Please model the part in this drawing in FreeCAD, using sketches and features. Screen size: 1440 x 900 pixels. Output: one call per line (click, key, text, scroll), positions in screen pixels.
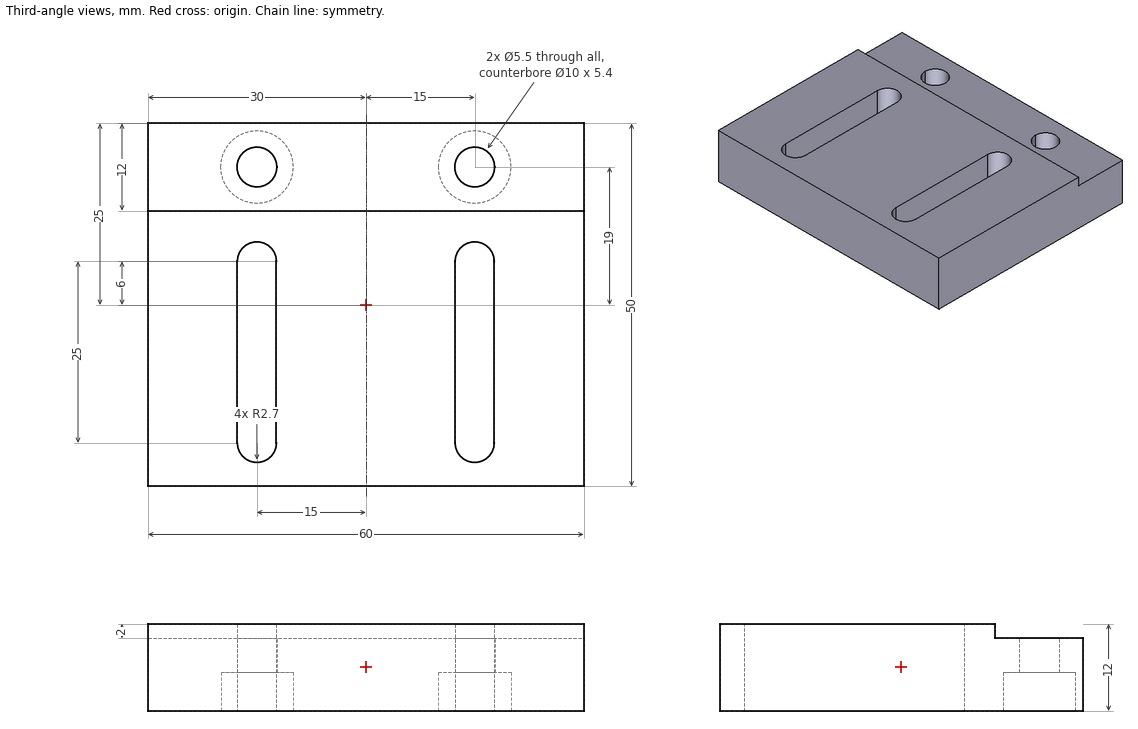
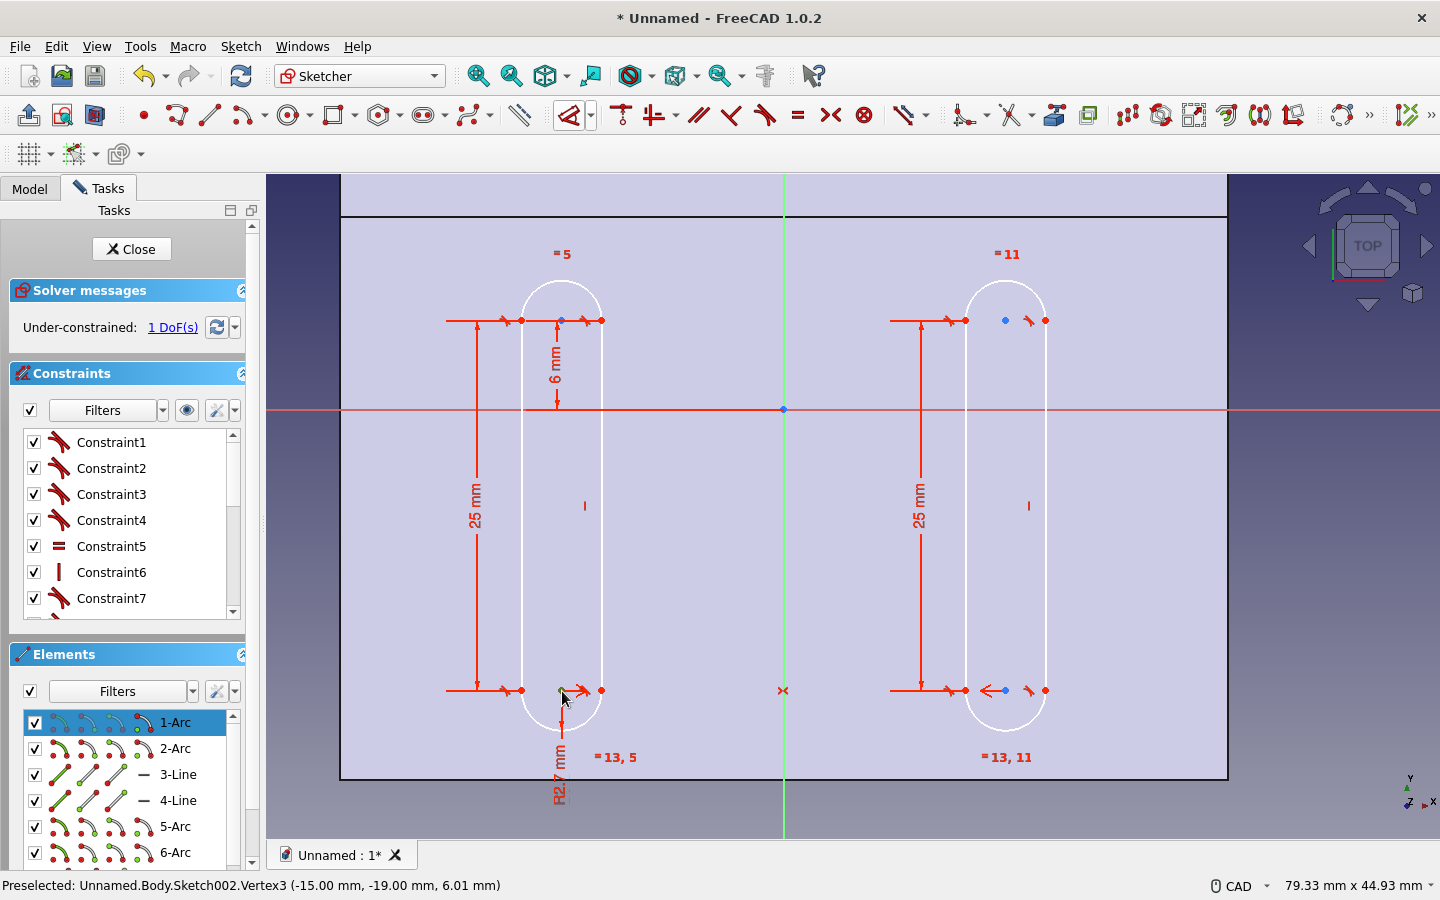
key(l)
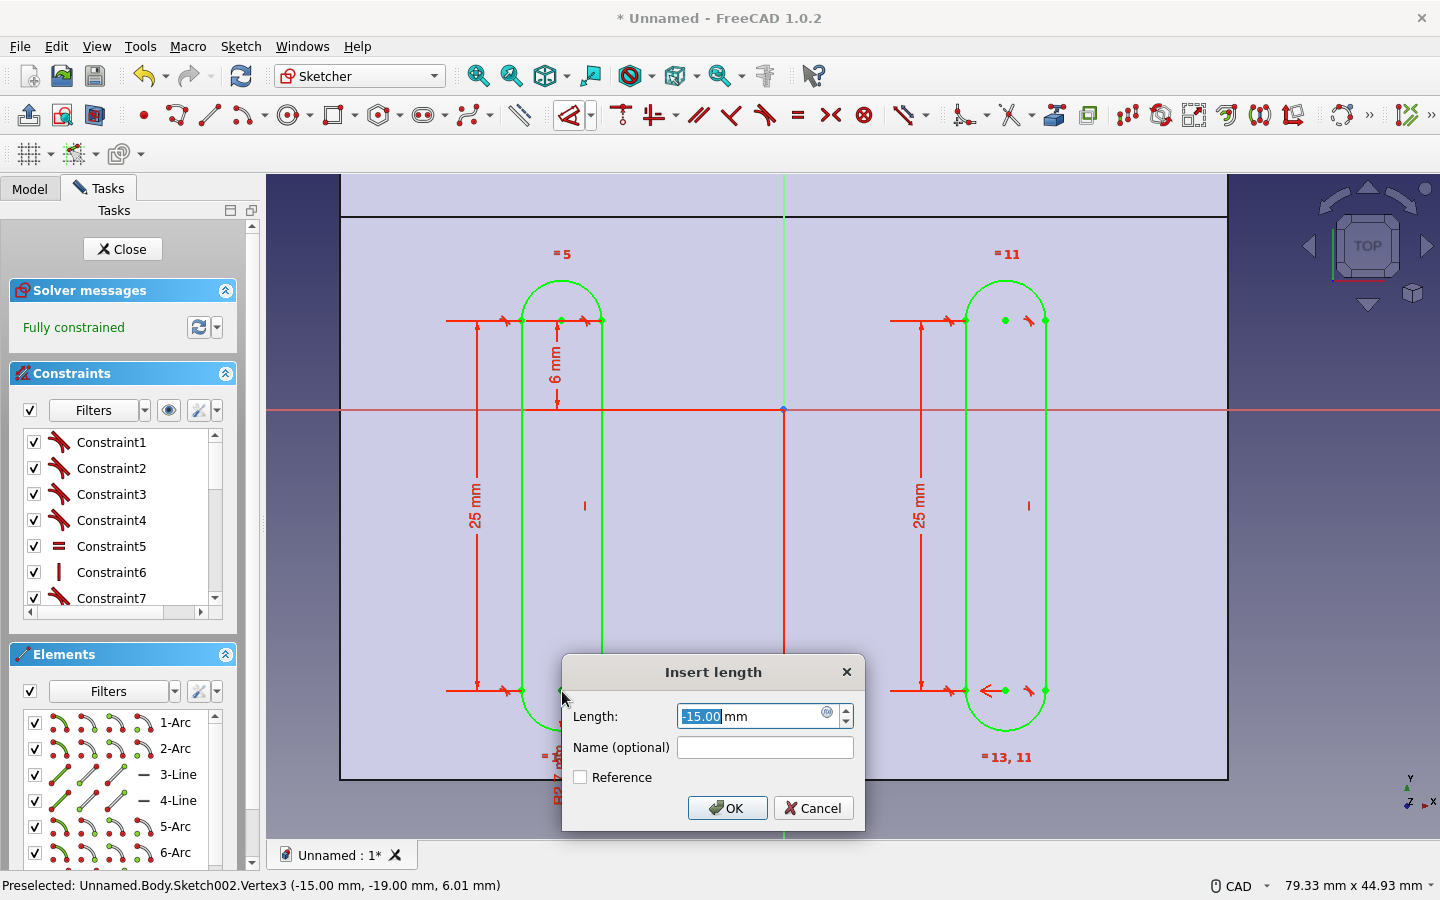
text(-15)
key(Return)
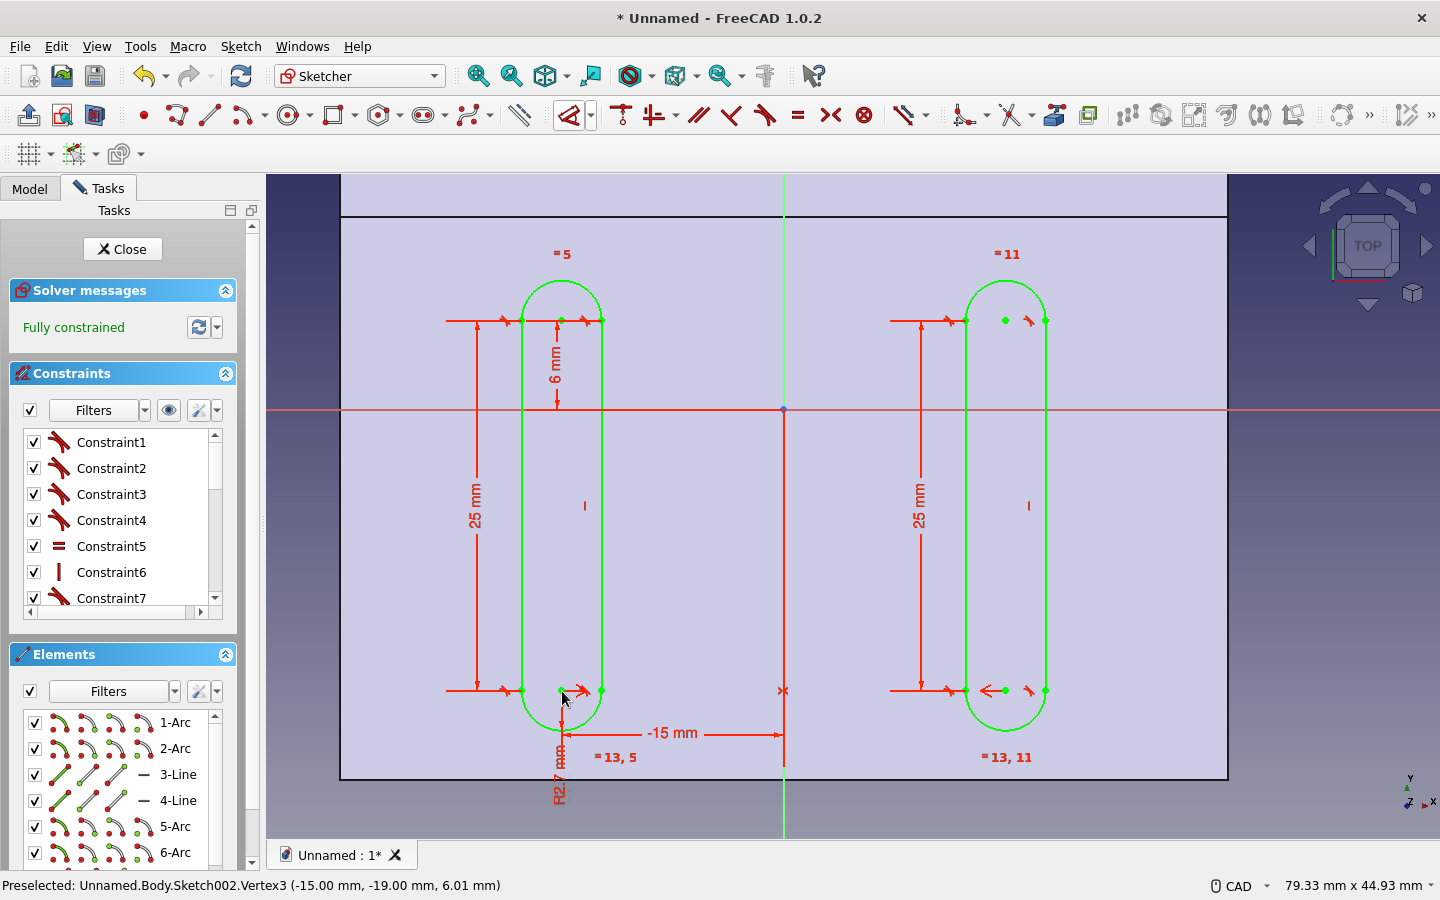
click(123, 249)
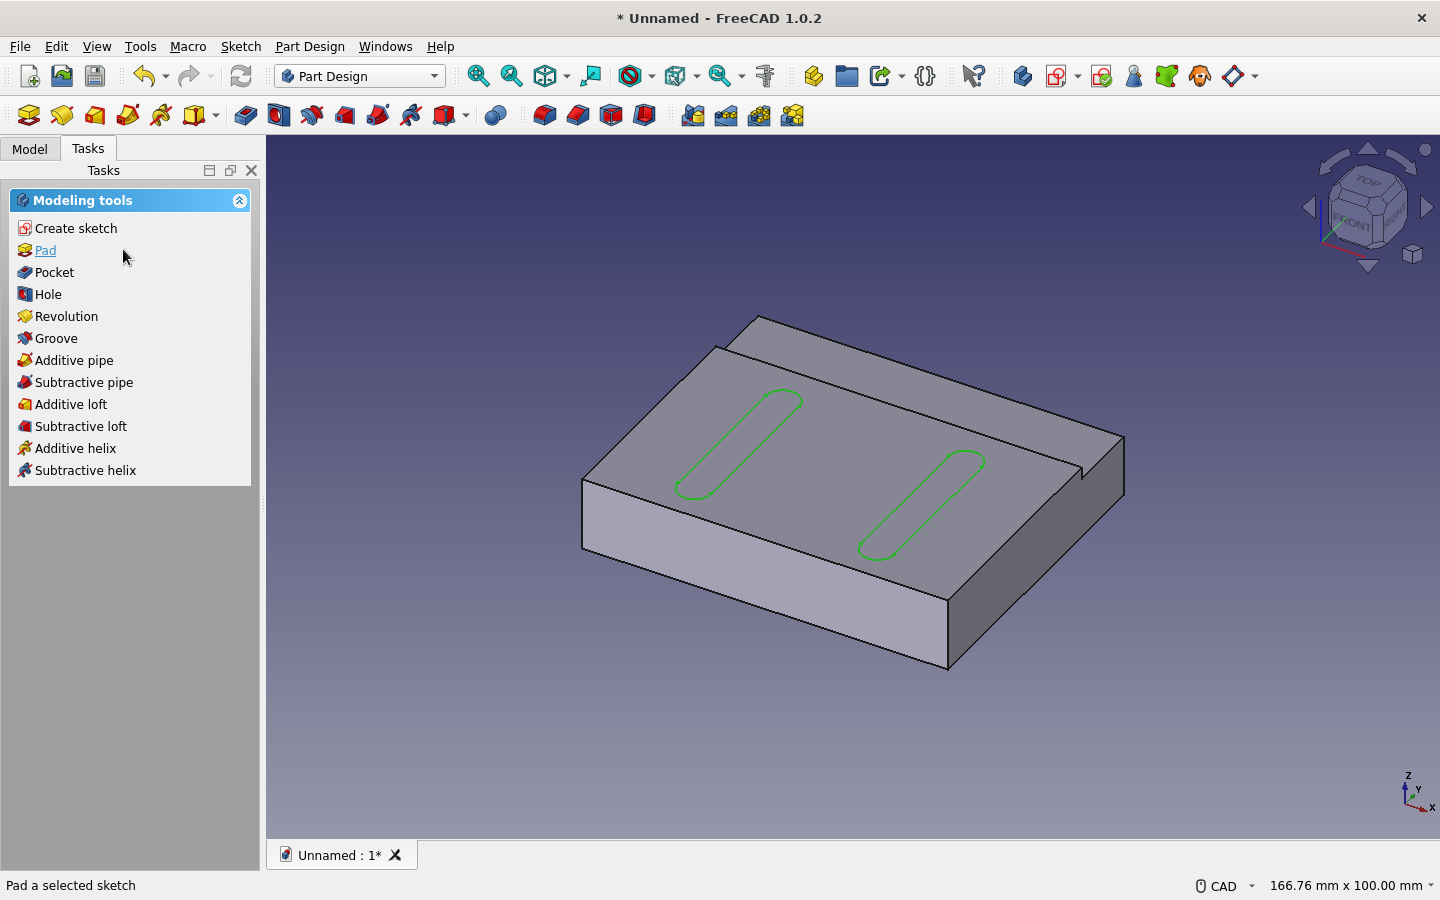
click(246, 116)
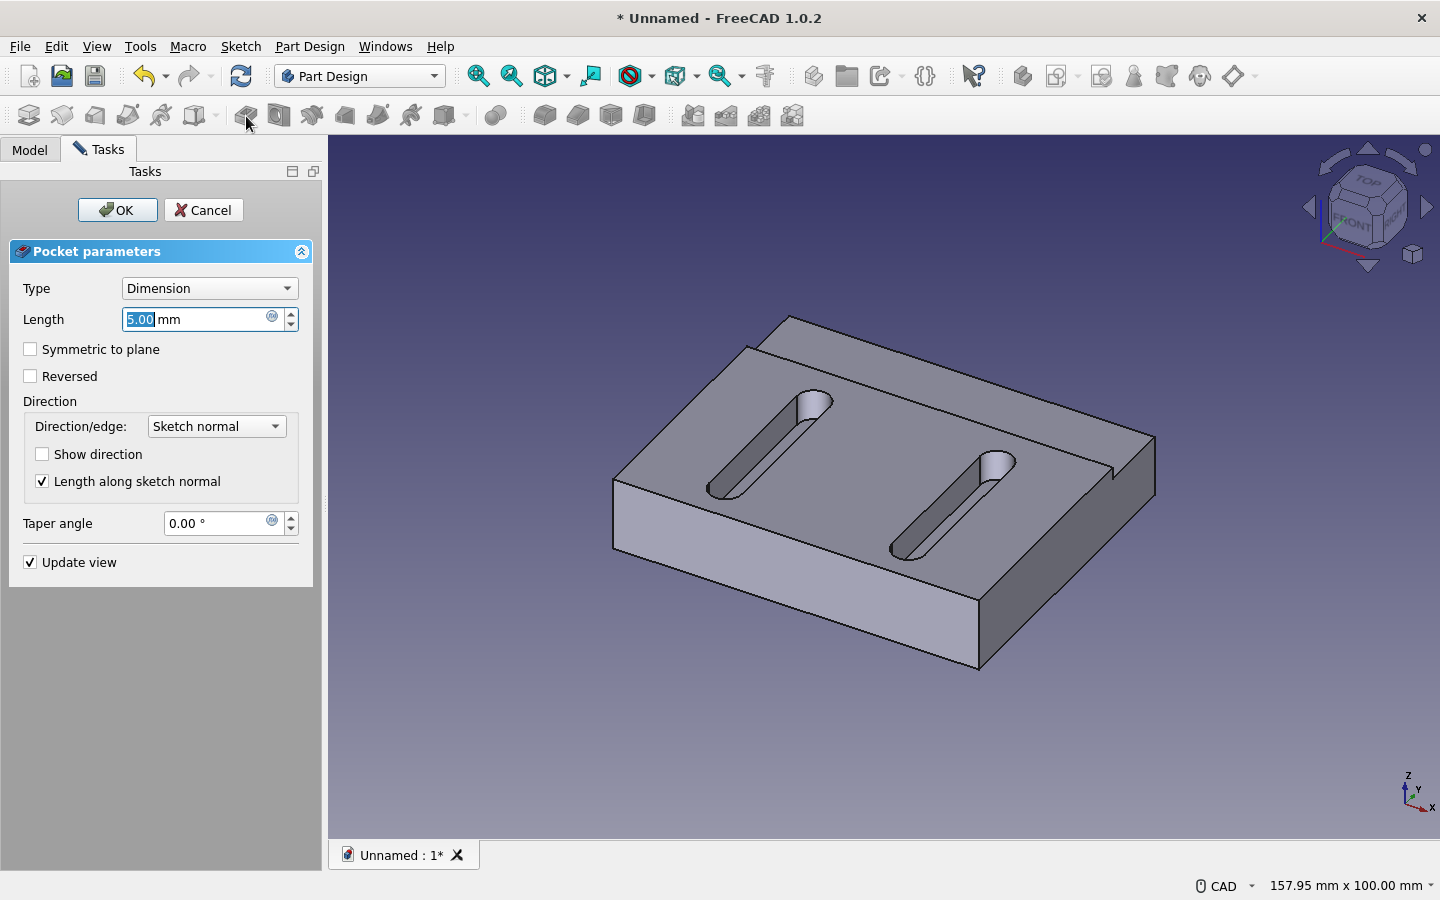
click(210, 288)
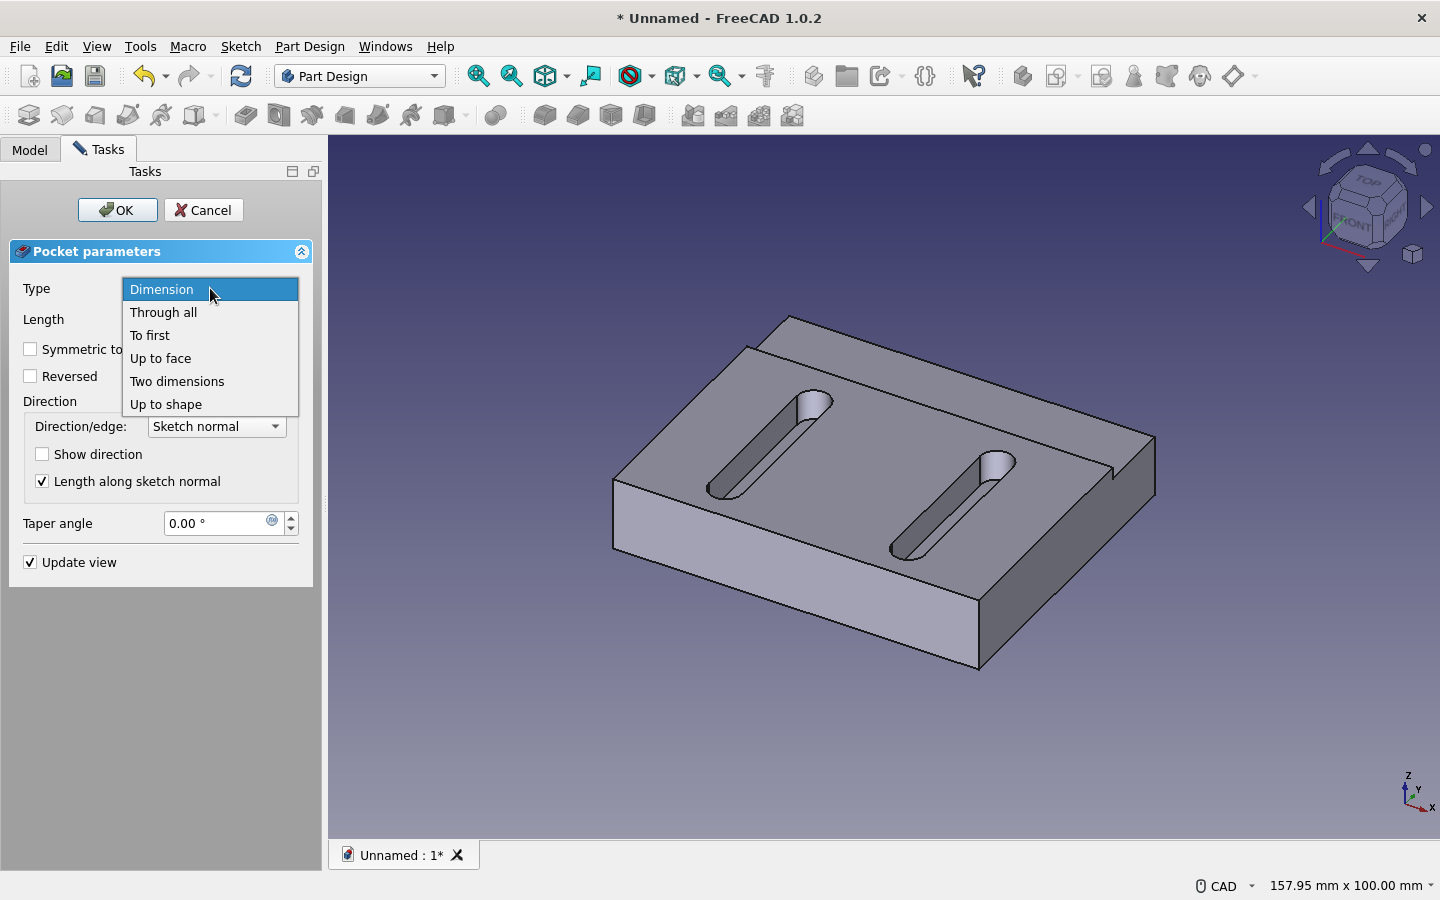
click(208, 312)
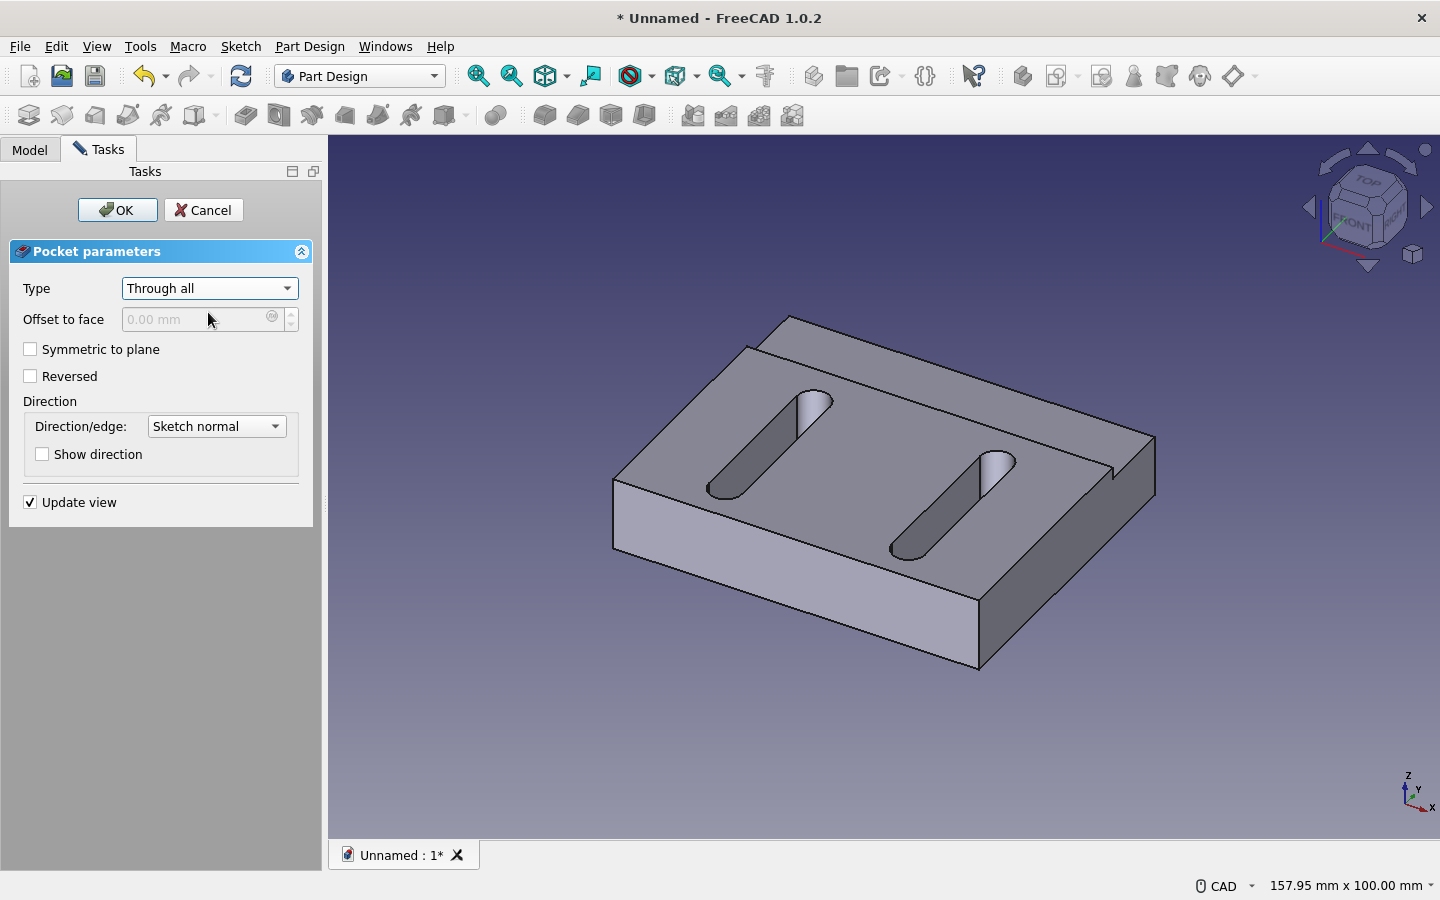
click(118, 210)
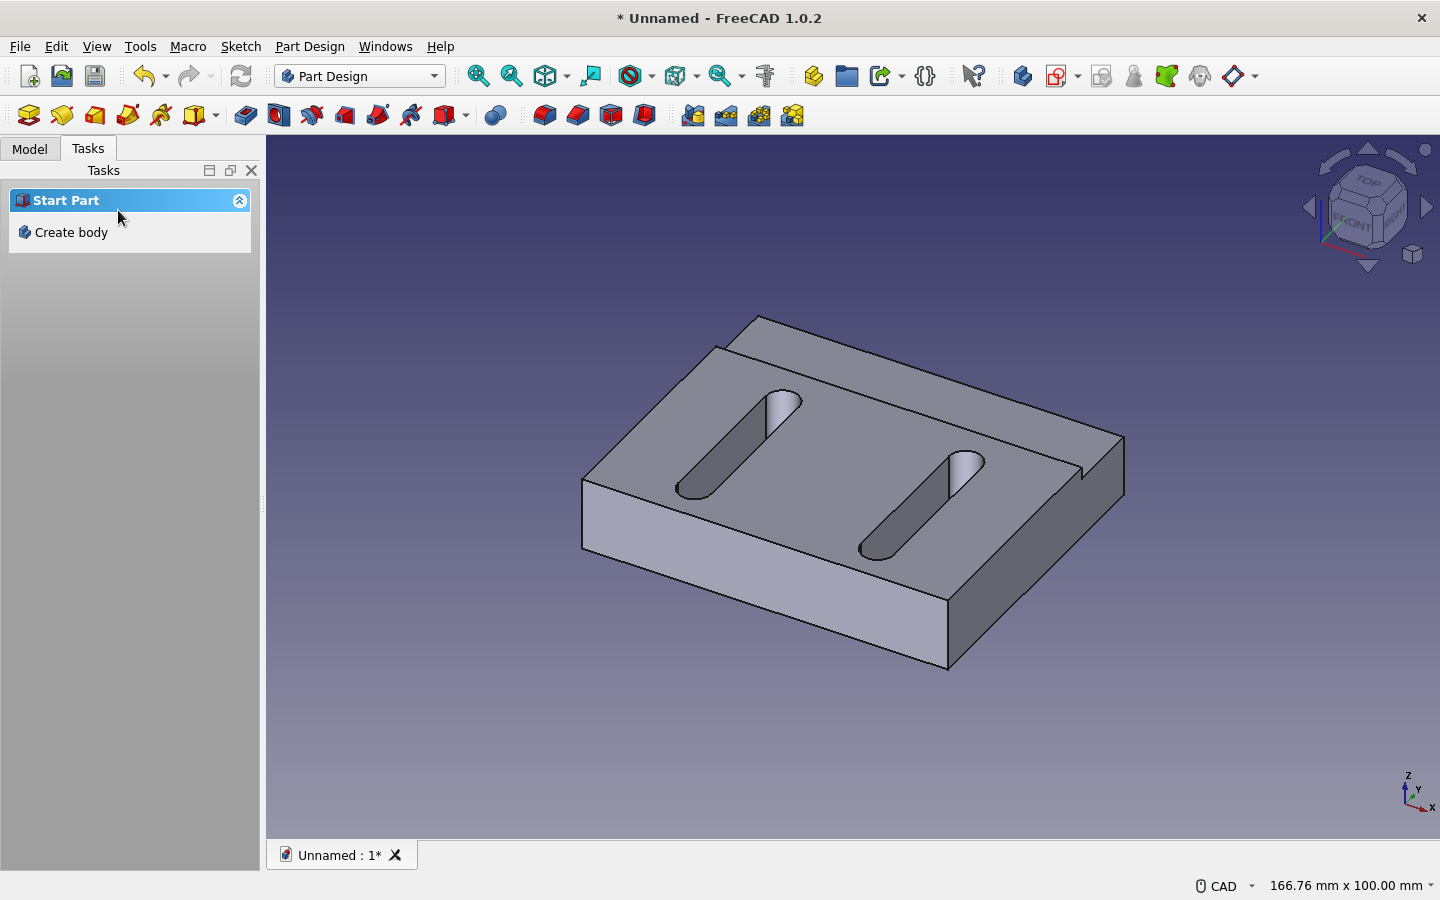
key(5)